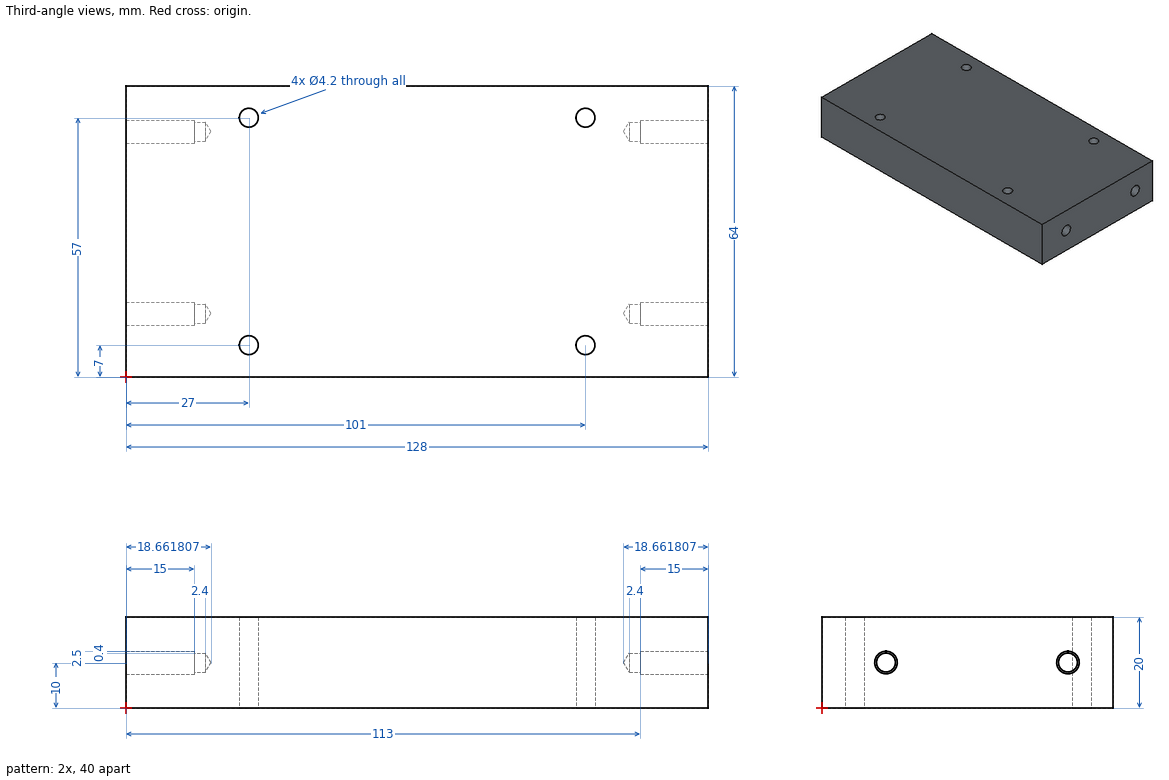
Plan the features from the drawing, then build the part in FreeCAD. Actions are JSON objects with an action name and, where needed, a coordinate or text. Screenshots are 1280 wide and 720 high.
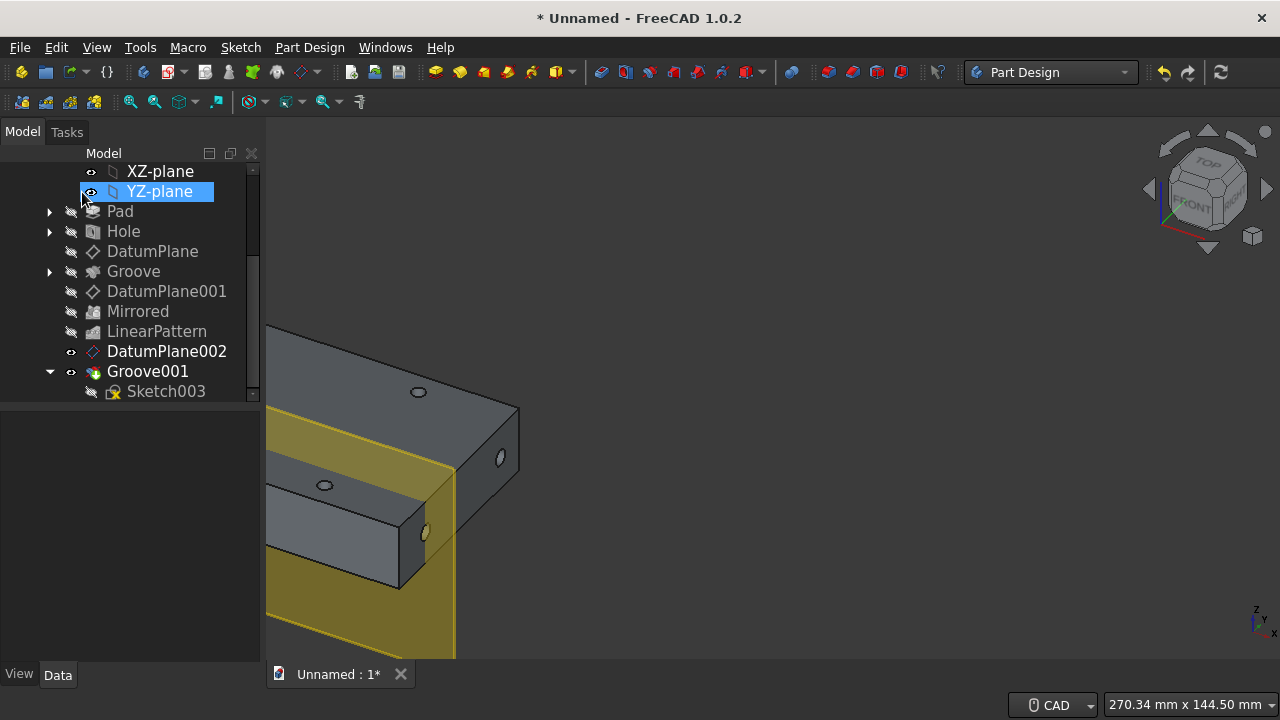
{"action": "left_click", "coordinate": [116, 352]}
{"action": "key", "text": "space"}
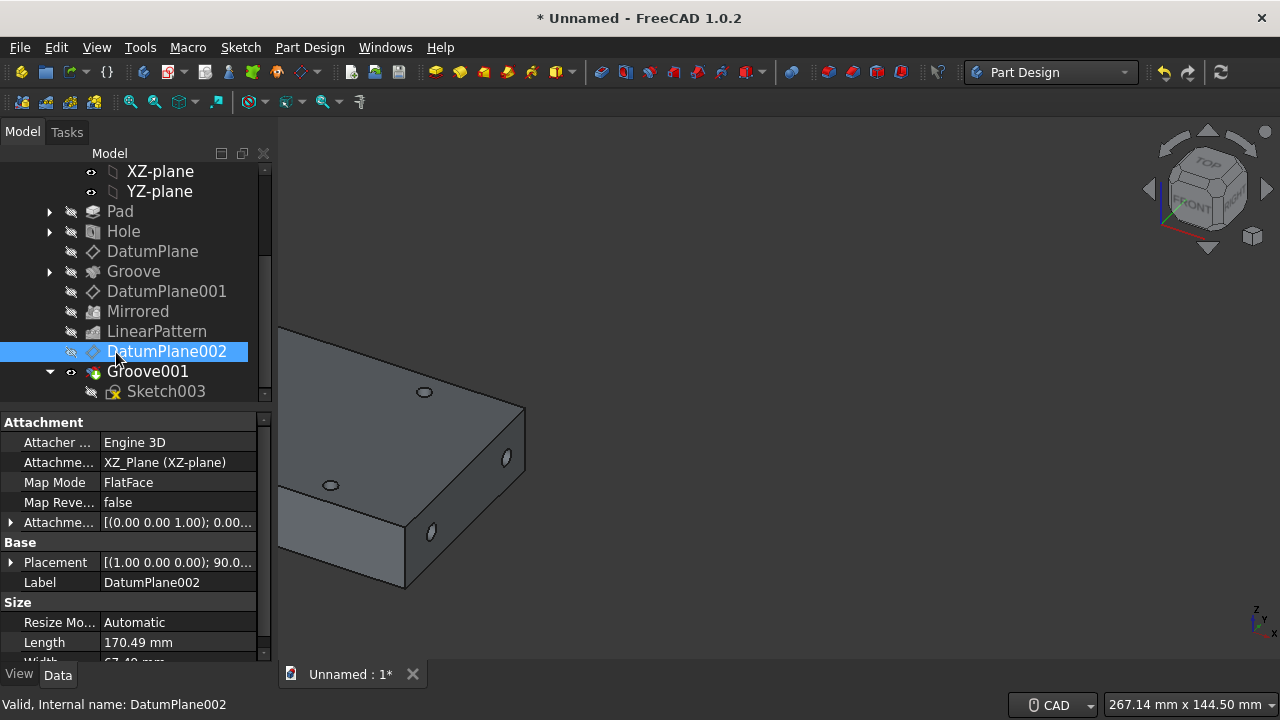
{"action": "left_click", "coordinate": [132, 102]}